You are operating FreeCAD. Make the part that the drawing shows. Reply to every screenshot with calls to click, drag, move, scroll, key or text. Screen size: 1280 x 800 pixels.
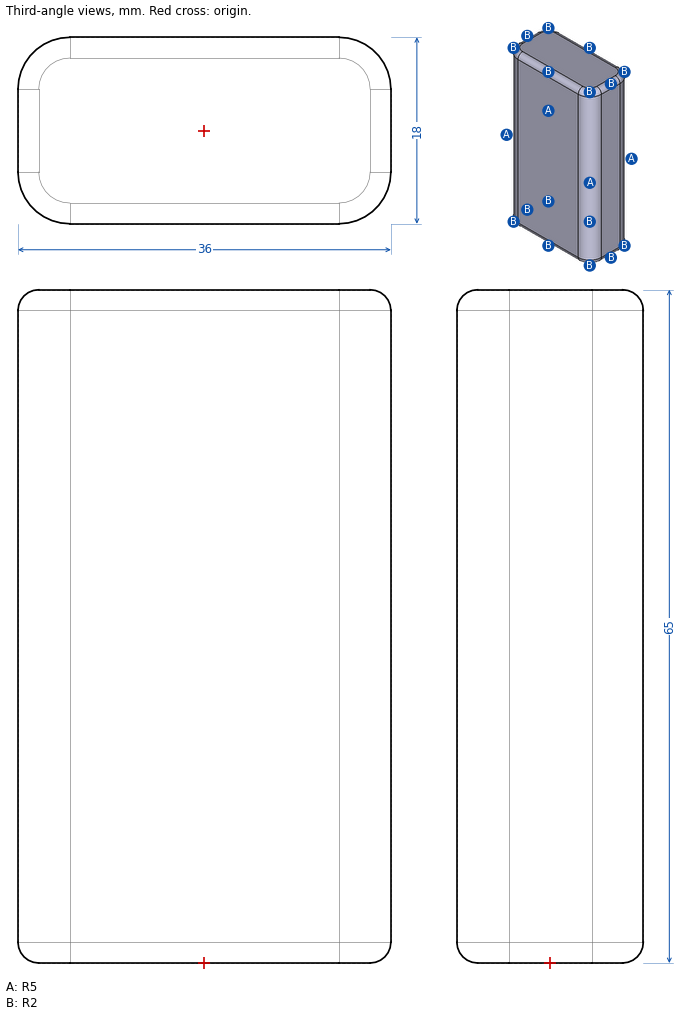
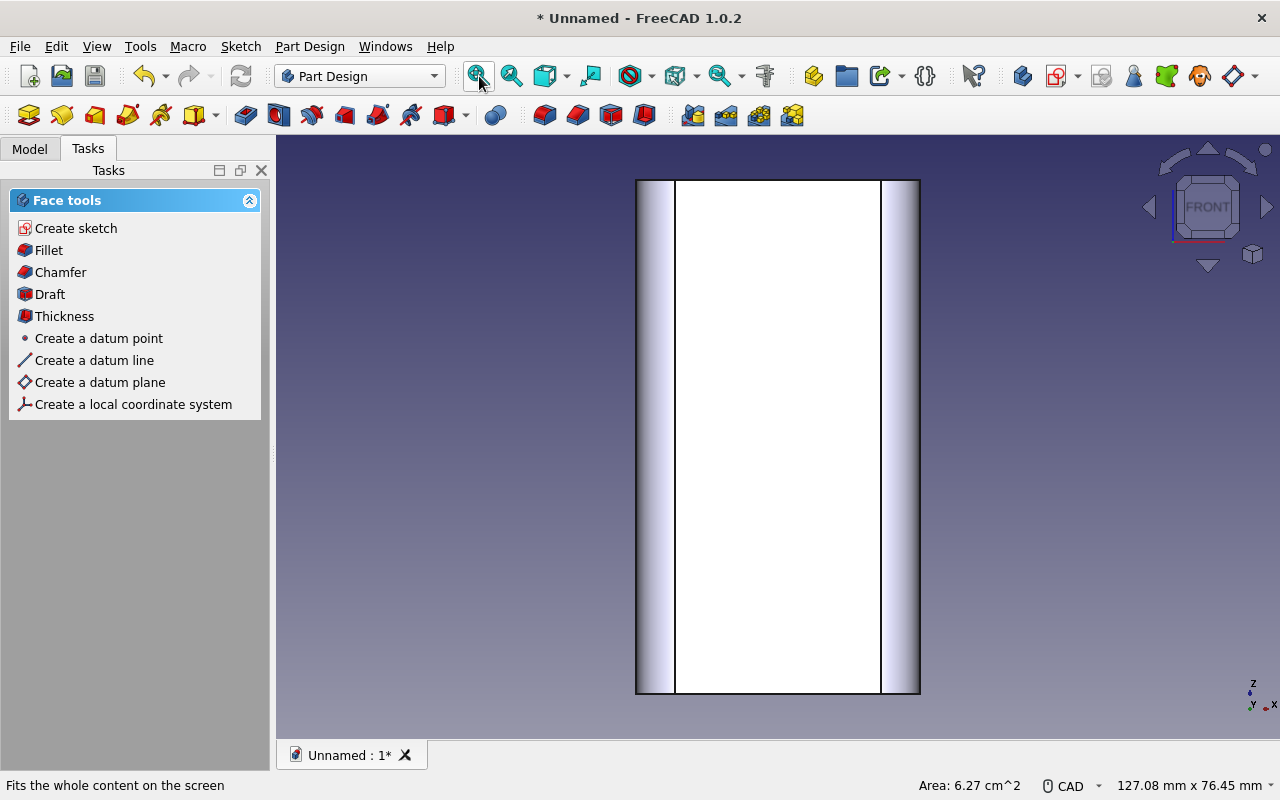
key(3)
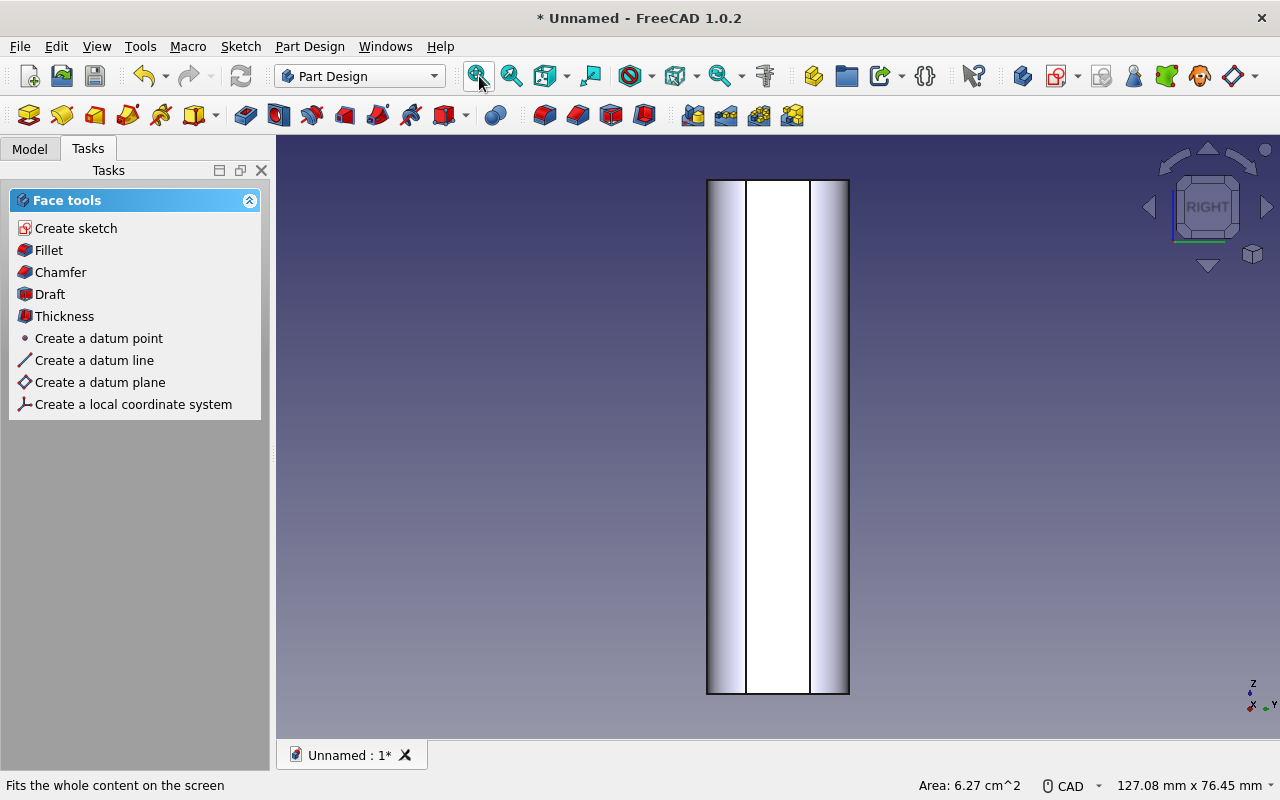
key(5)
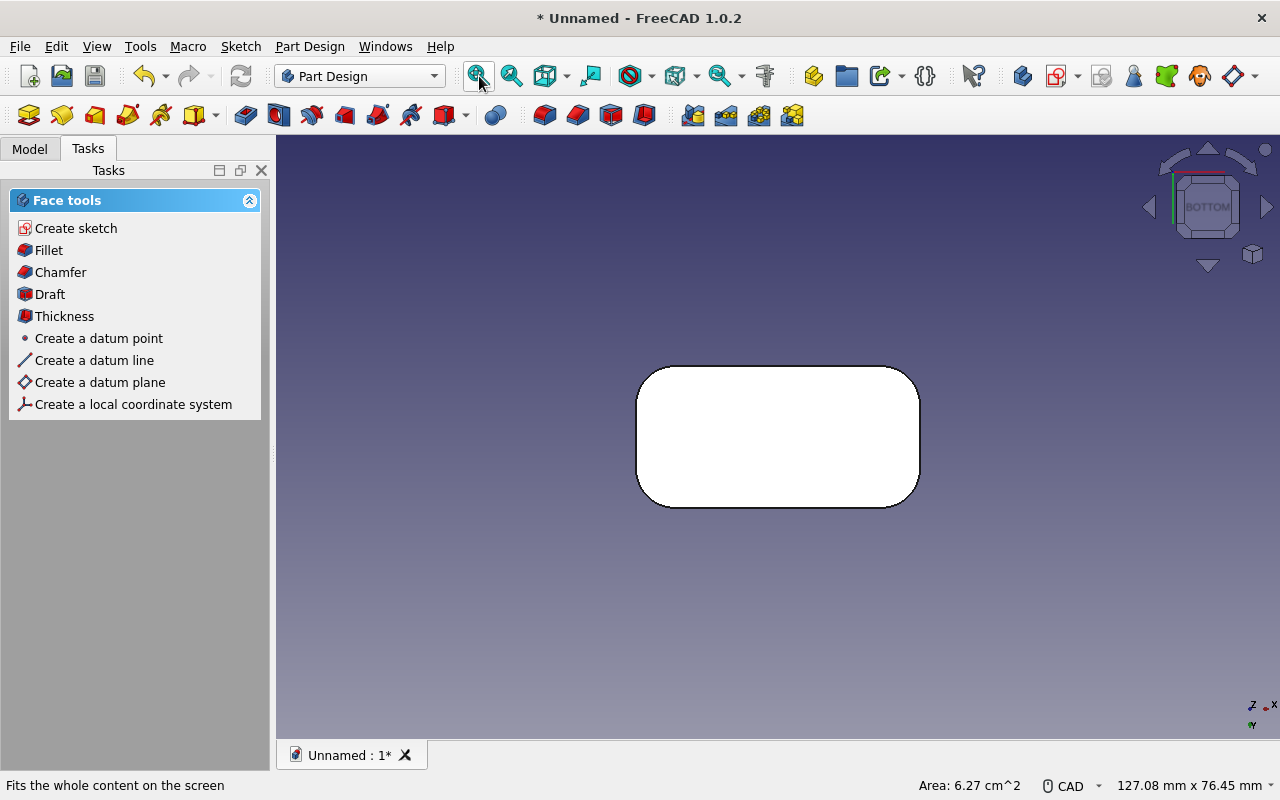
click(479, 76)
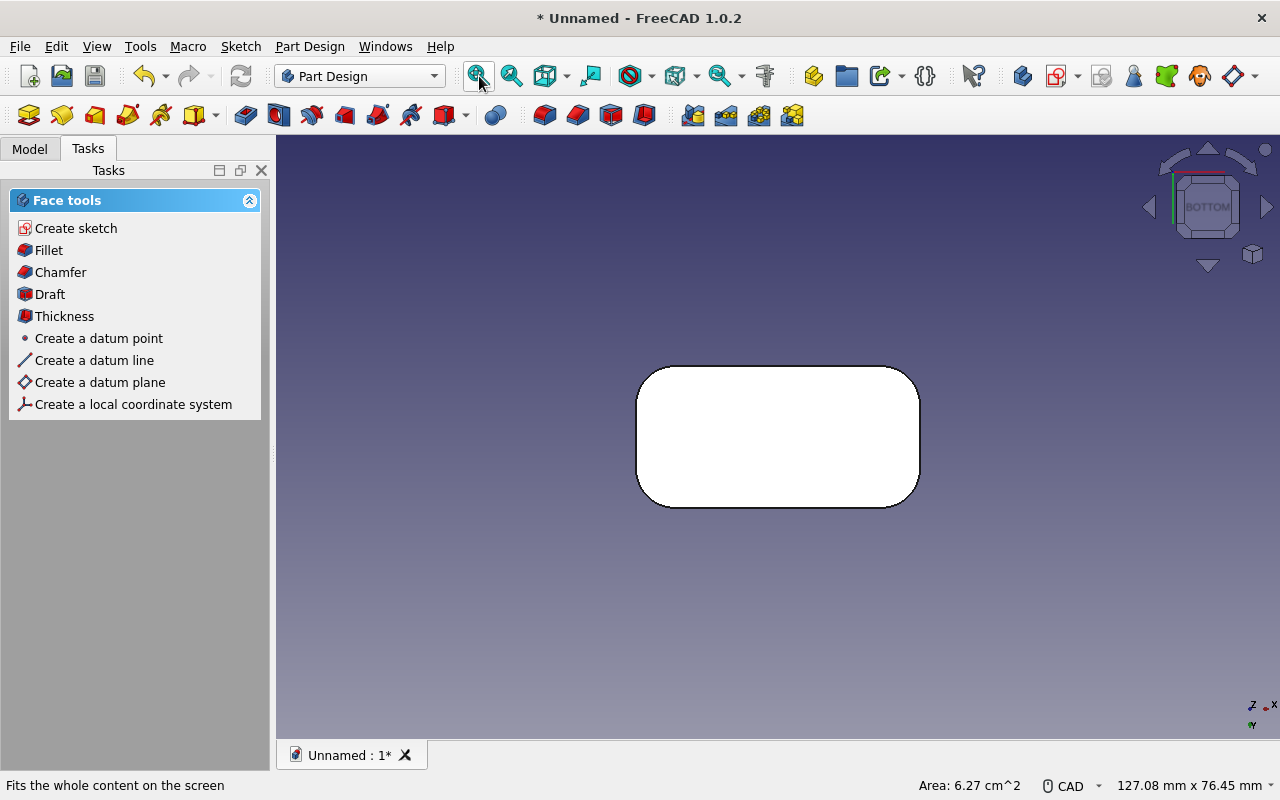
click(819, 436, ctrl)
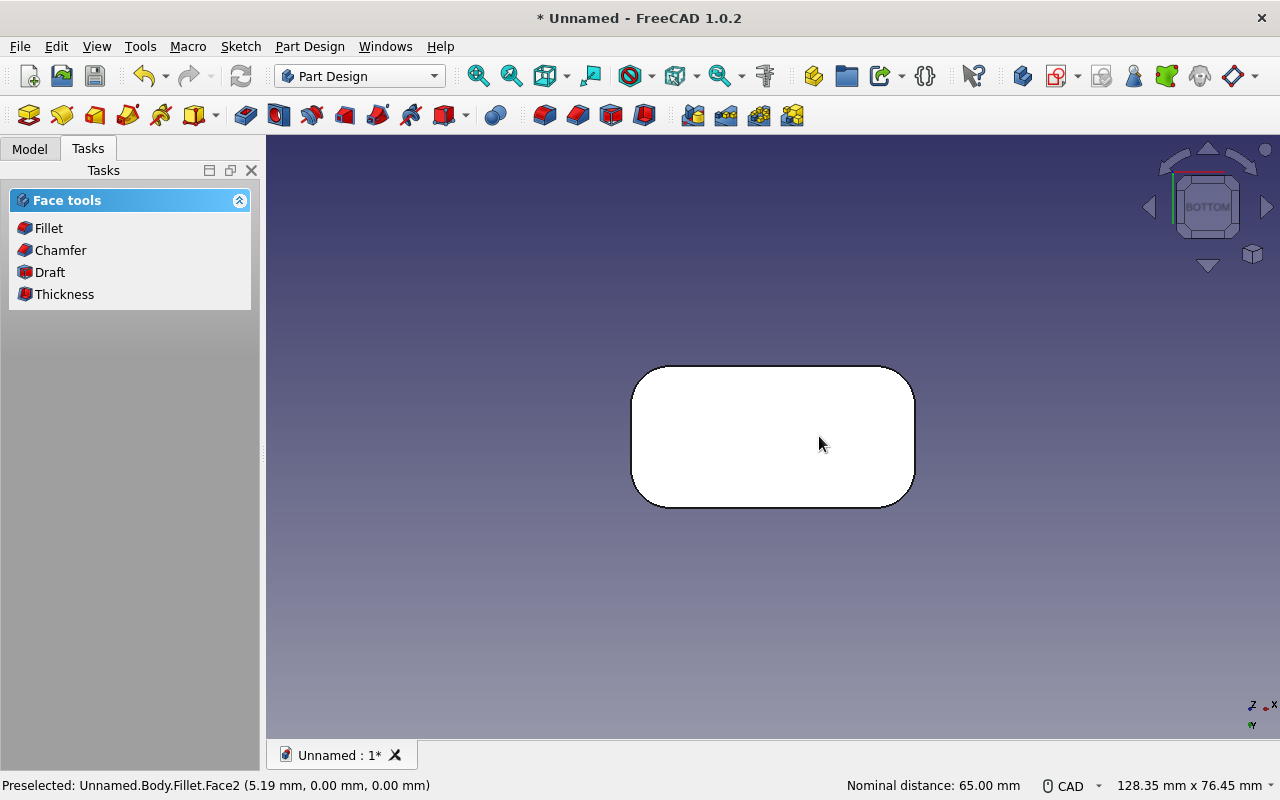
click(545, 116)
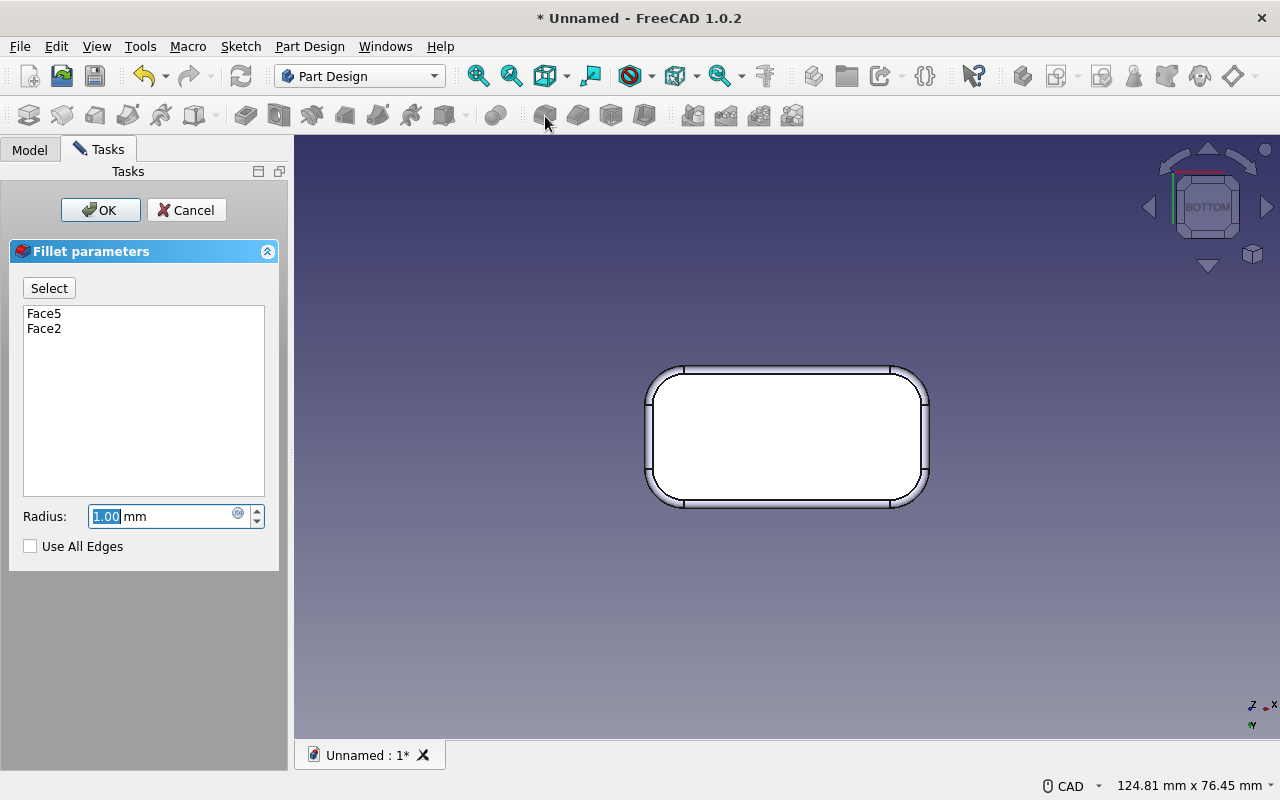
text(2)
key(Tab)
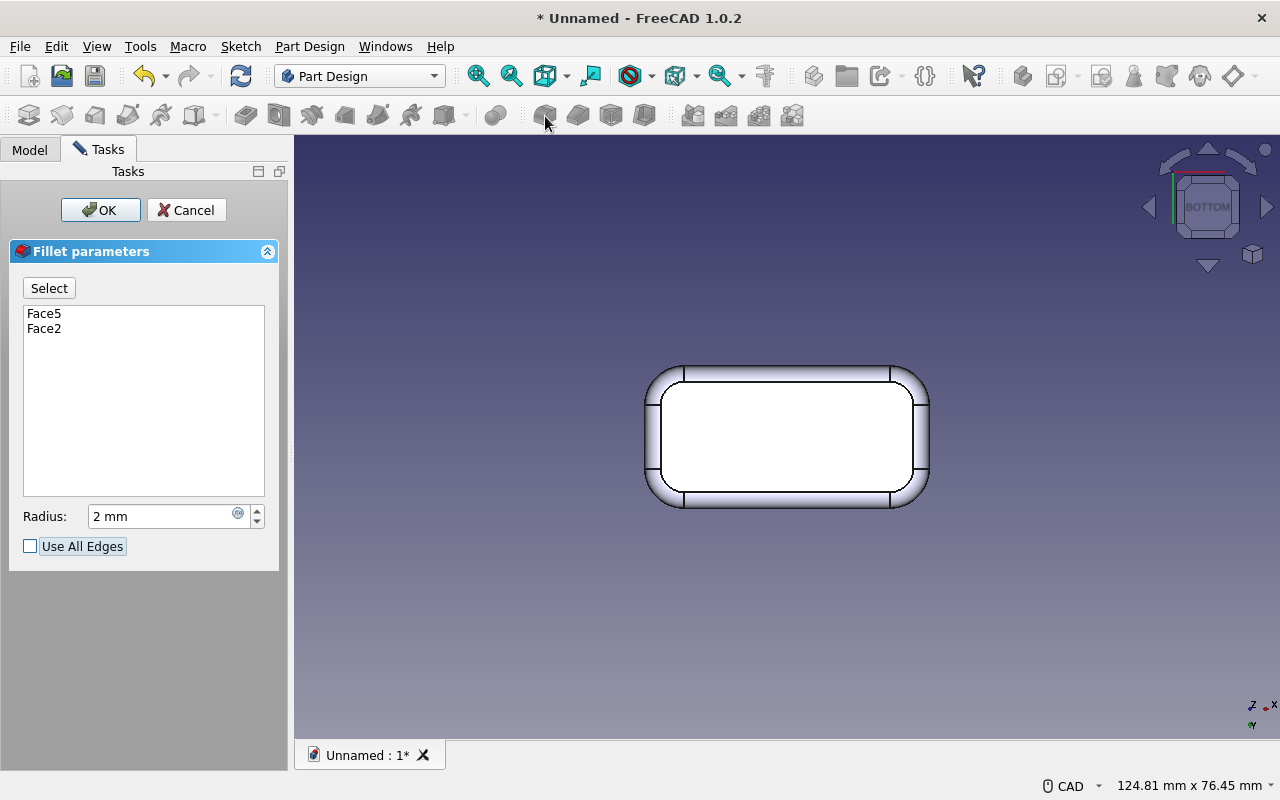
click(101, 210)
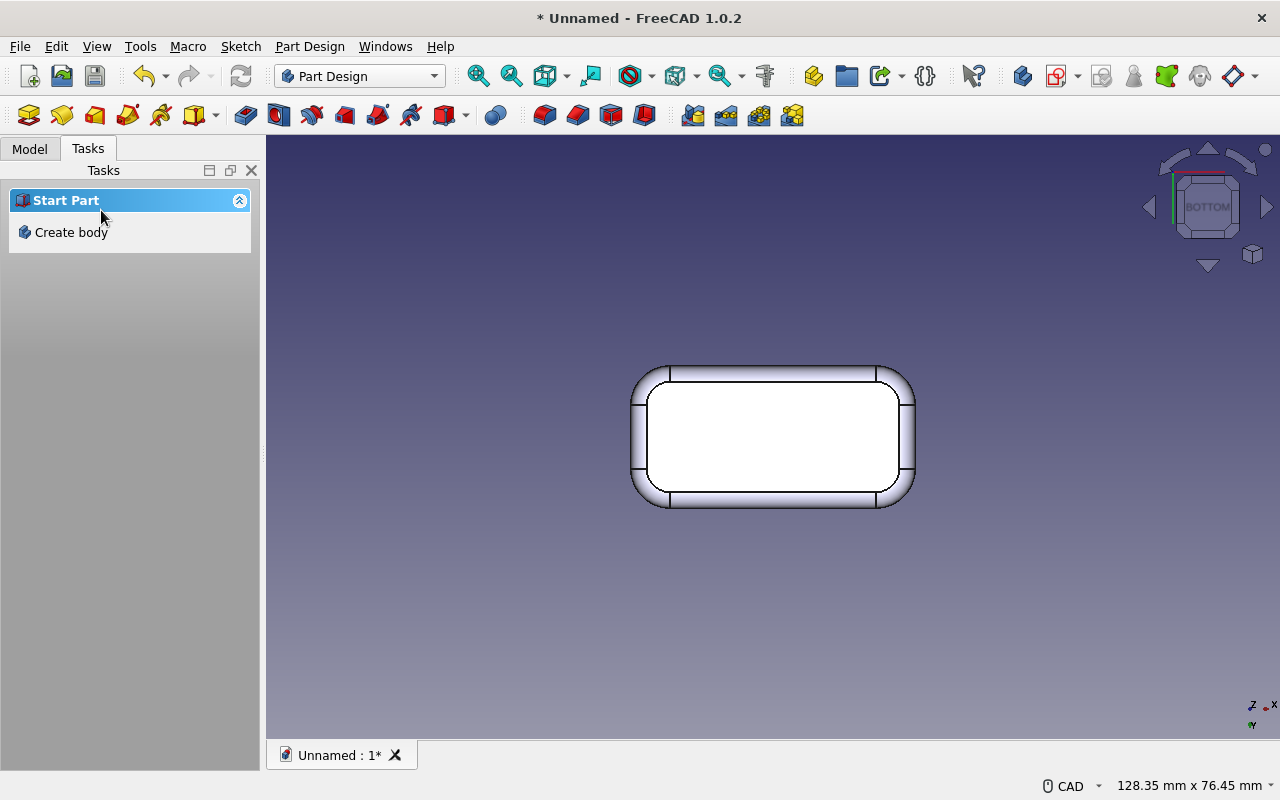
key(0)